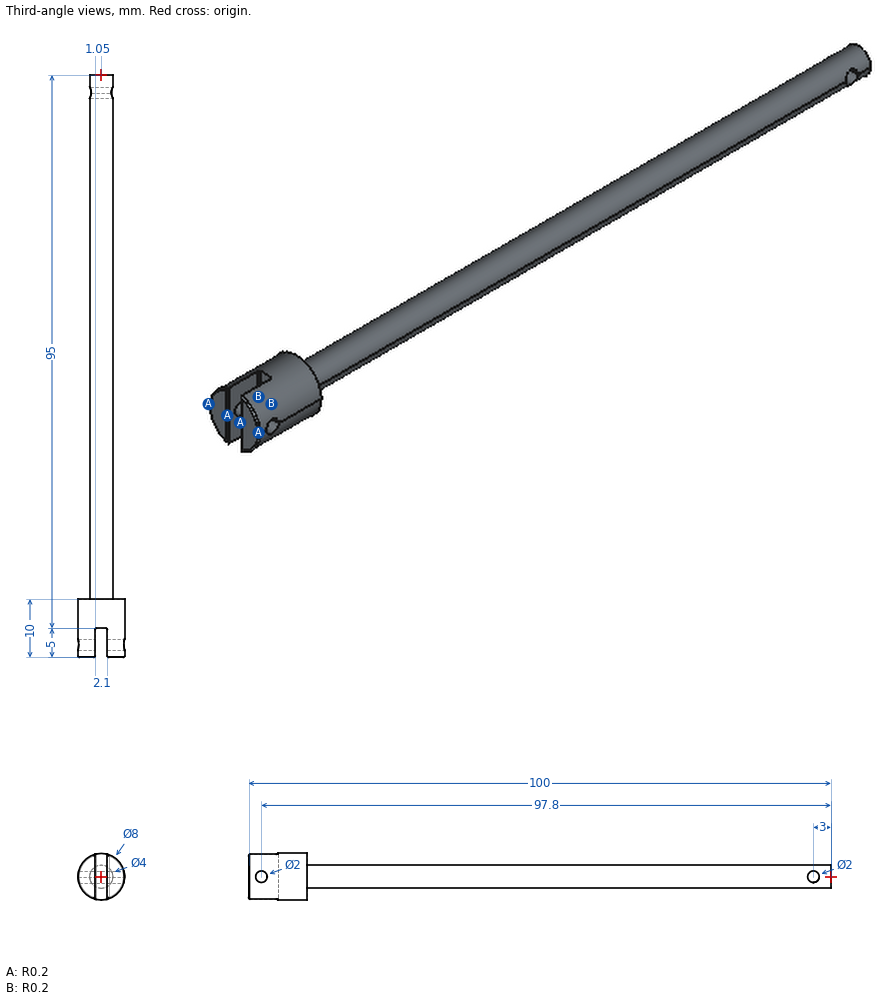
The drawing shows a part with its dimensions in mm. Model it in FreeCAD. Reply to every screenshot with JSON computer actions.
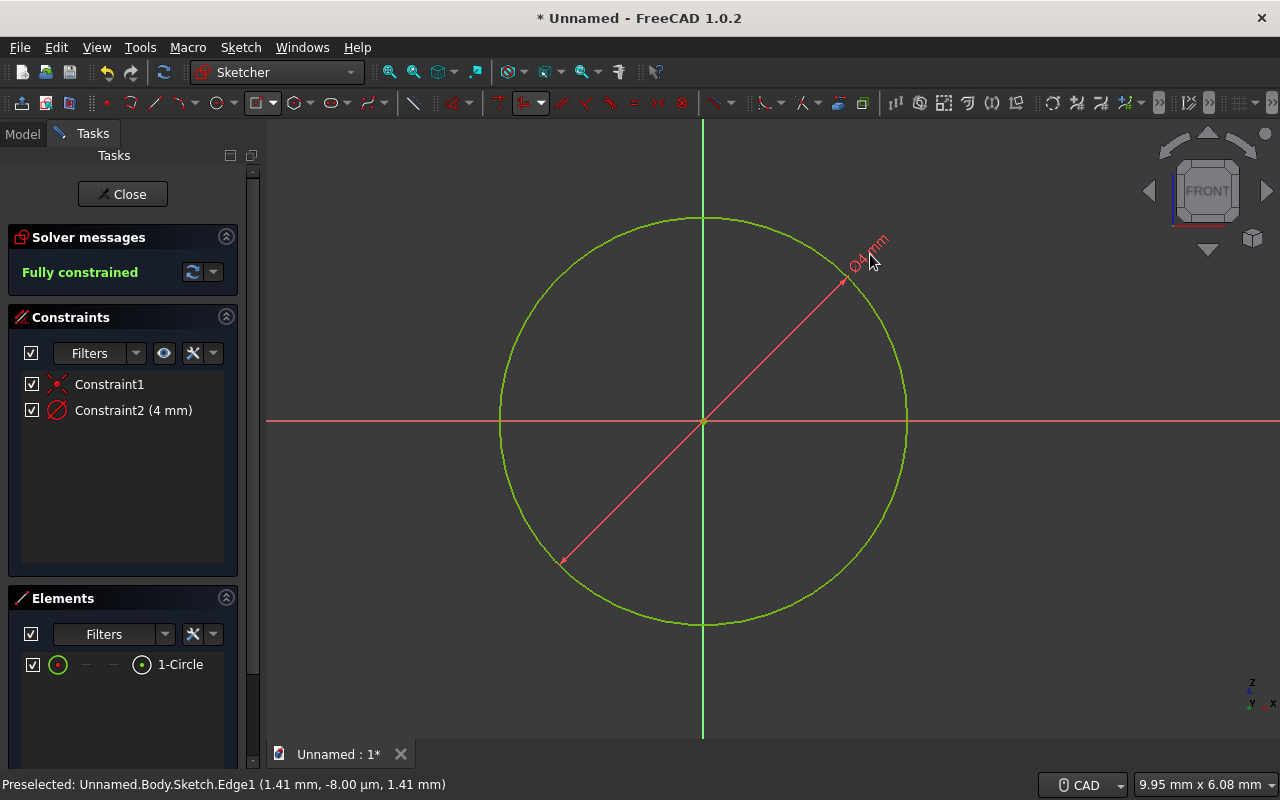
{"action": "left_click", "coordinate": [123, 194]}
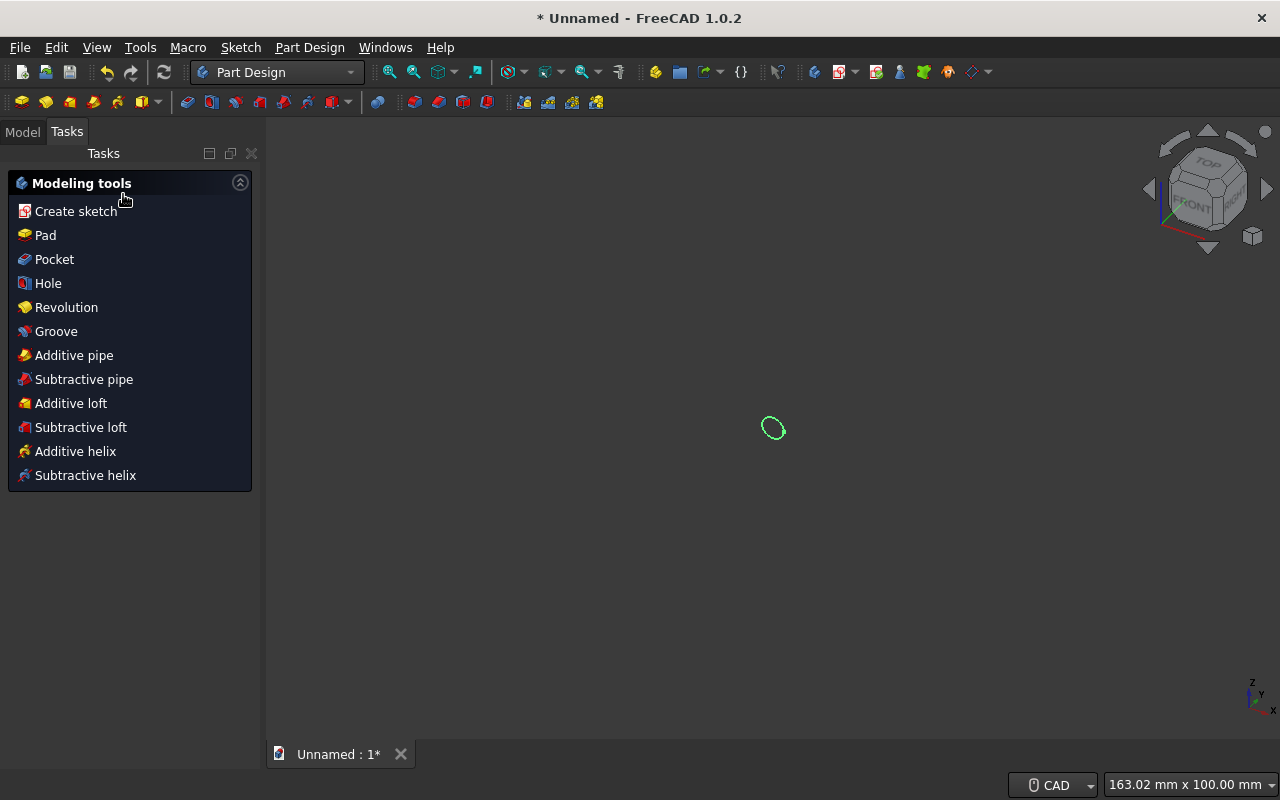
{"action": "left_click", "coordinate": [22, 102]}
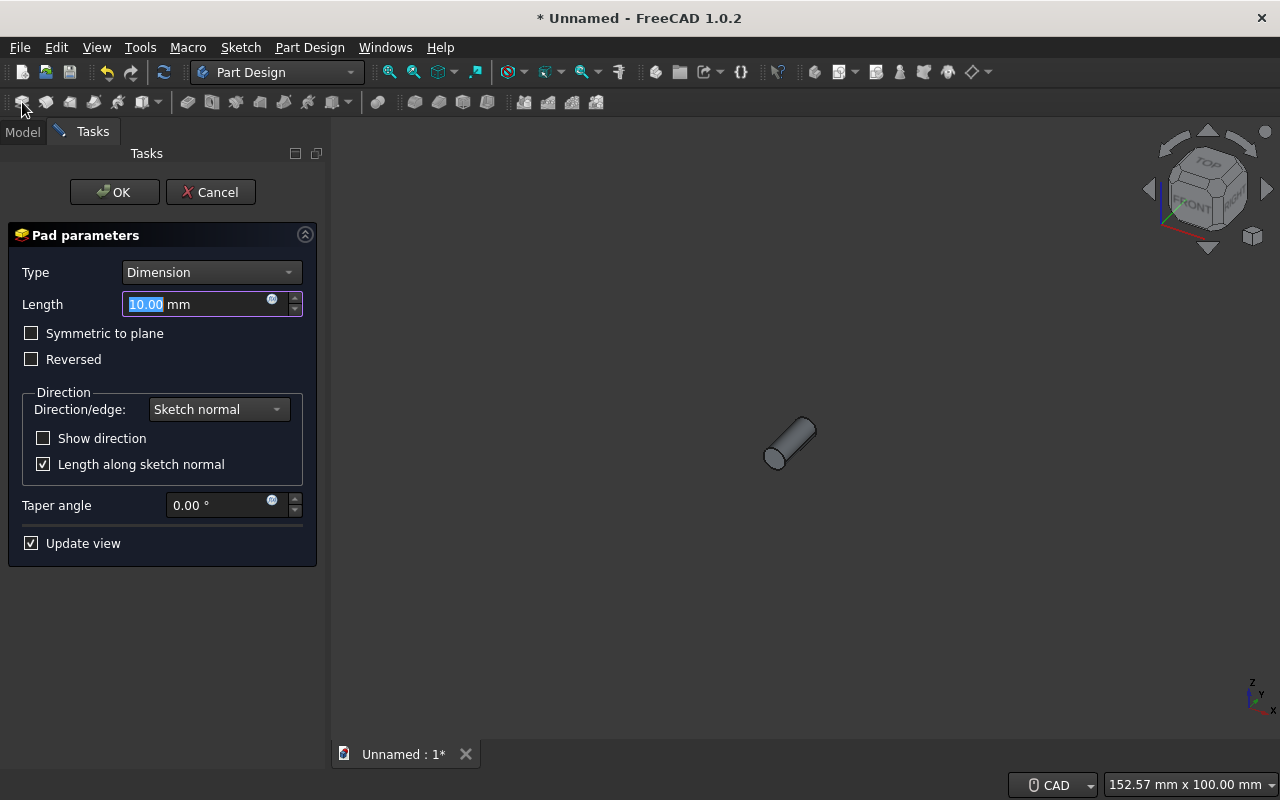
{"action": "type", "text": "100"}
{"action": "key", "text": "Tab"}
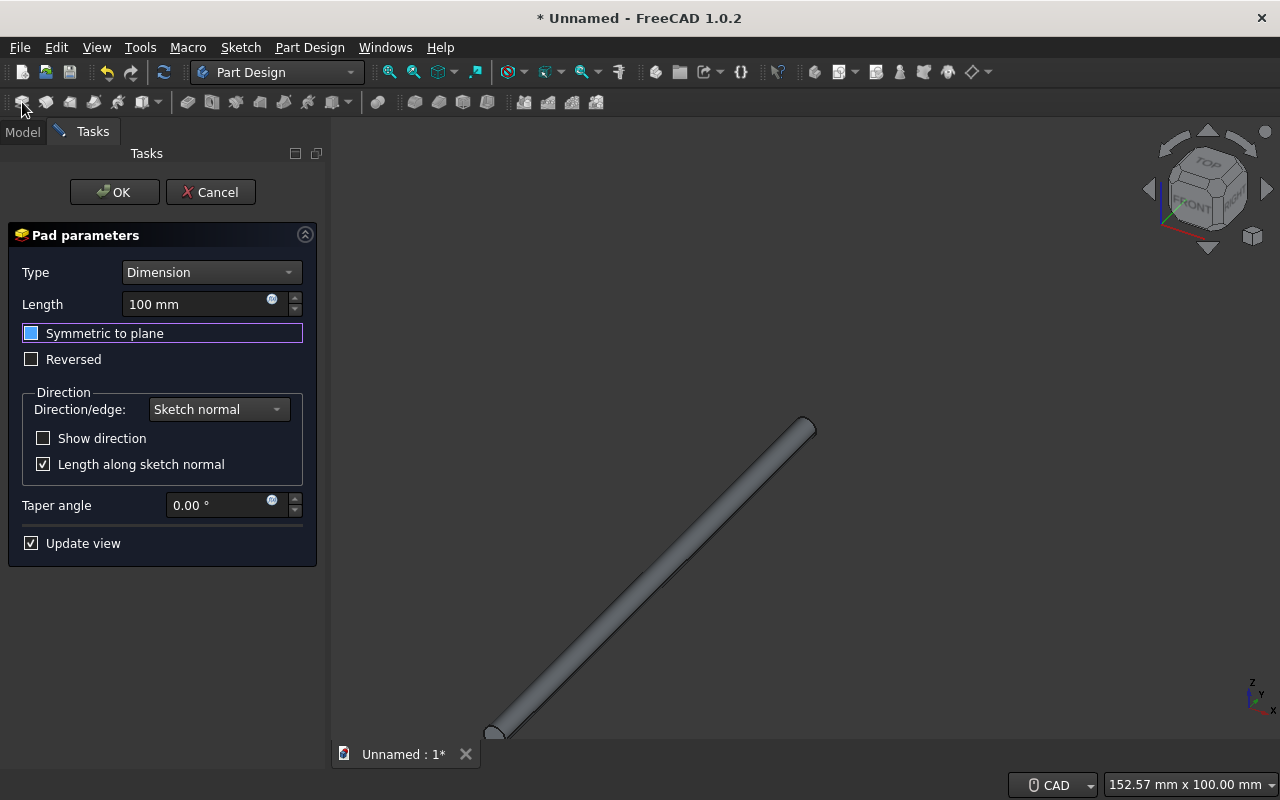
{"action": "left_click", "coordinate": [115, 192]}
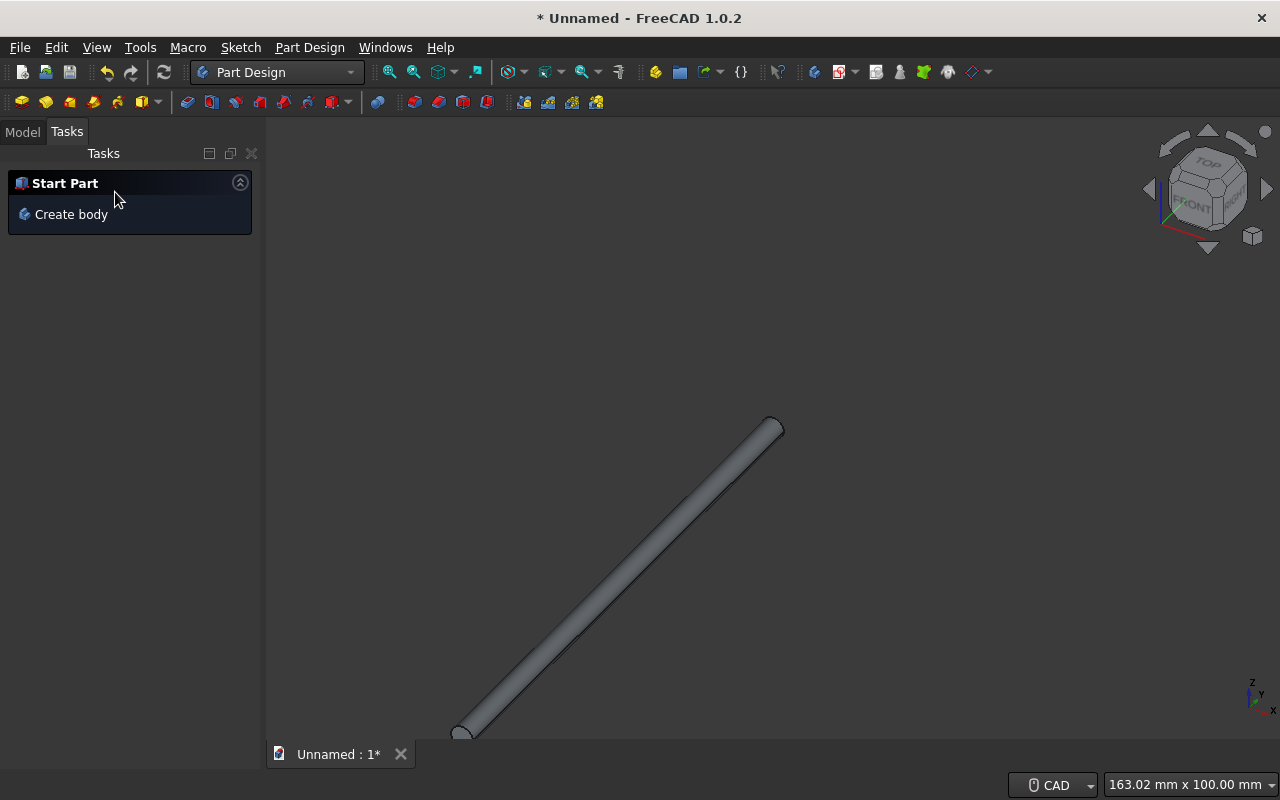
{"action": "left_click", "coordinate": [390, 72]}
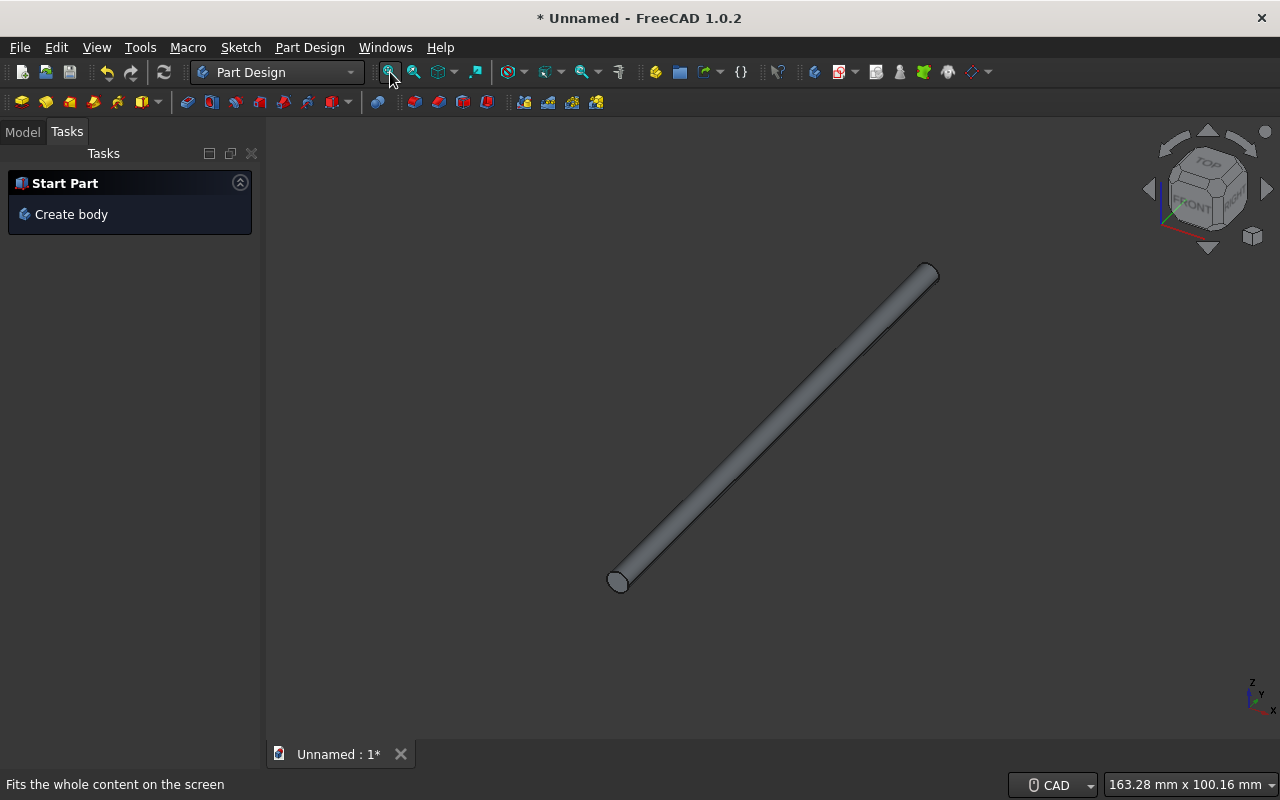
{"action": "left_click", "coordinate": [618, 584]}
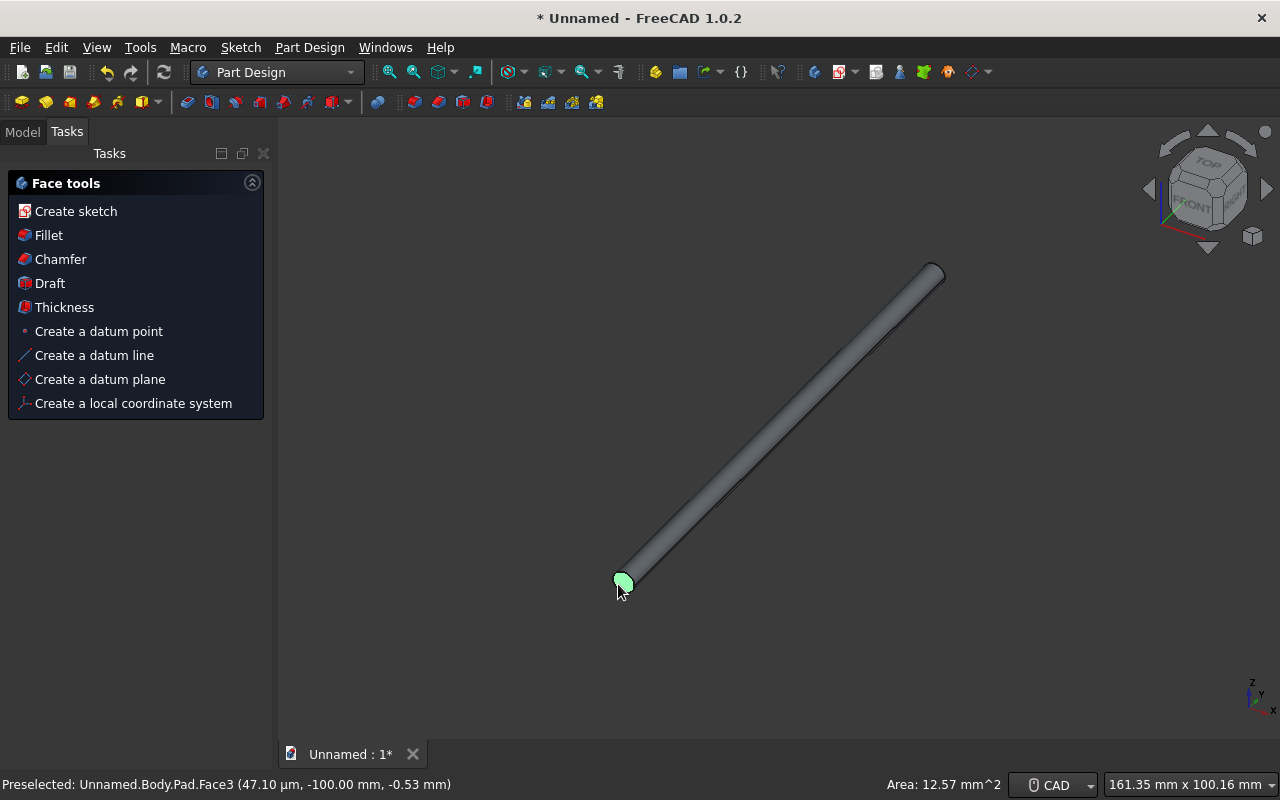
{"action": "left_click", "coordinate": [840, 72]}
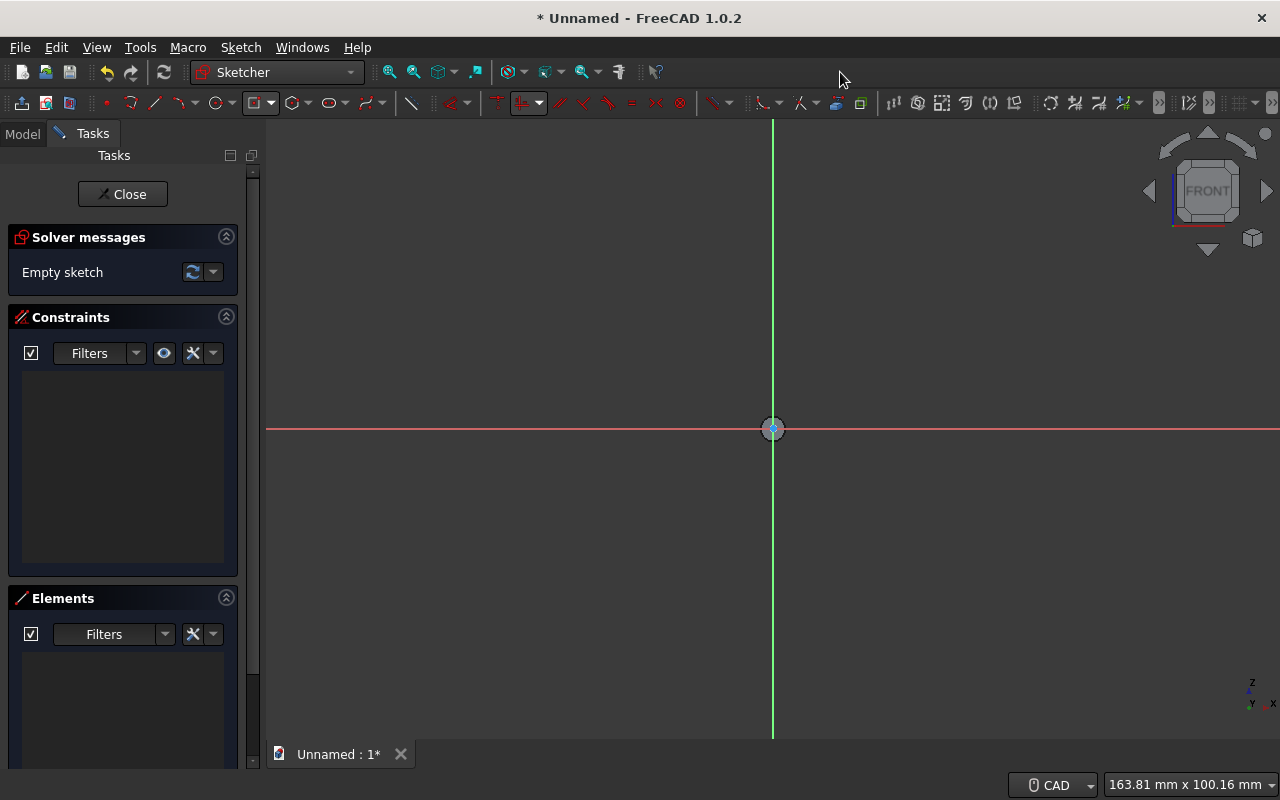
{"action": "scroll", "coordinate": [784, 429], "scroll_direction": "up", "scroll_amount": 10}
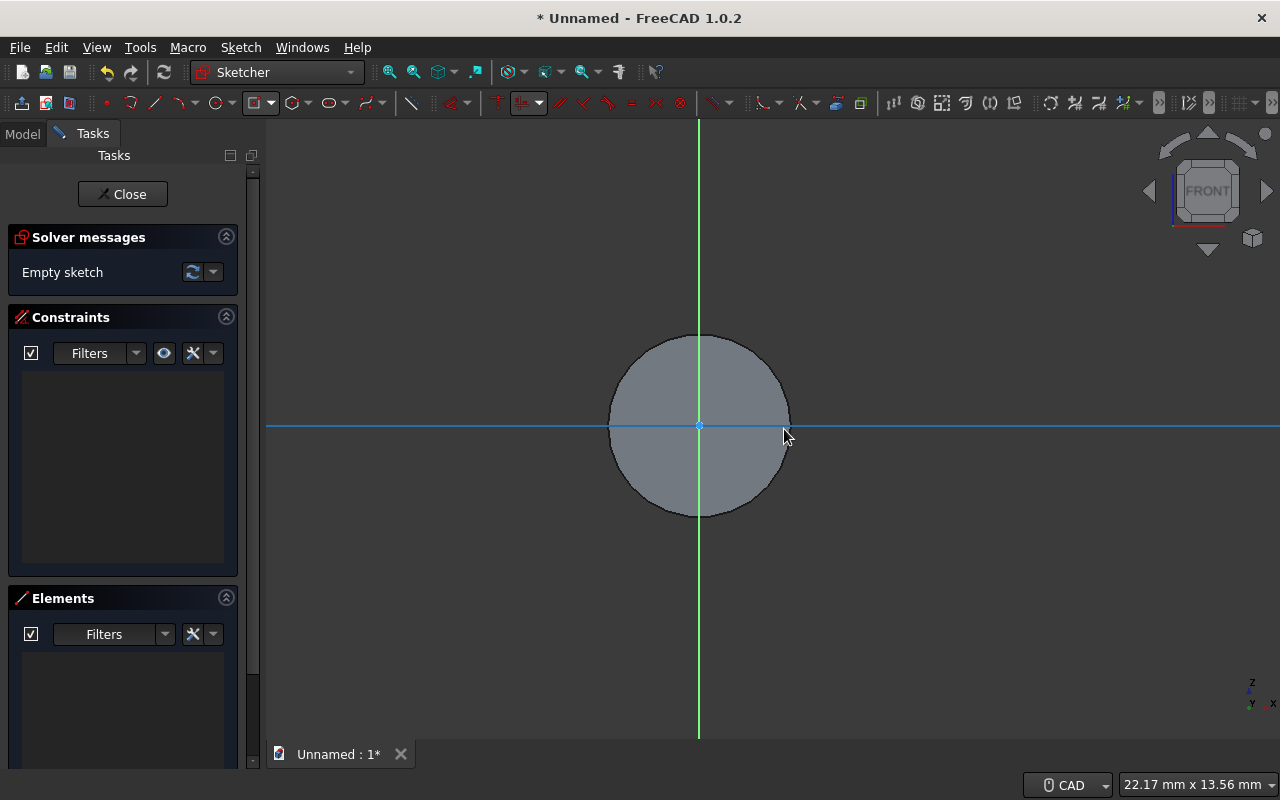
{"action": "left_click", "coordinate": [216, 104]}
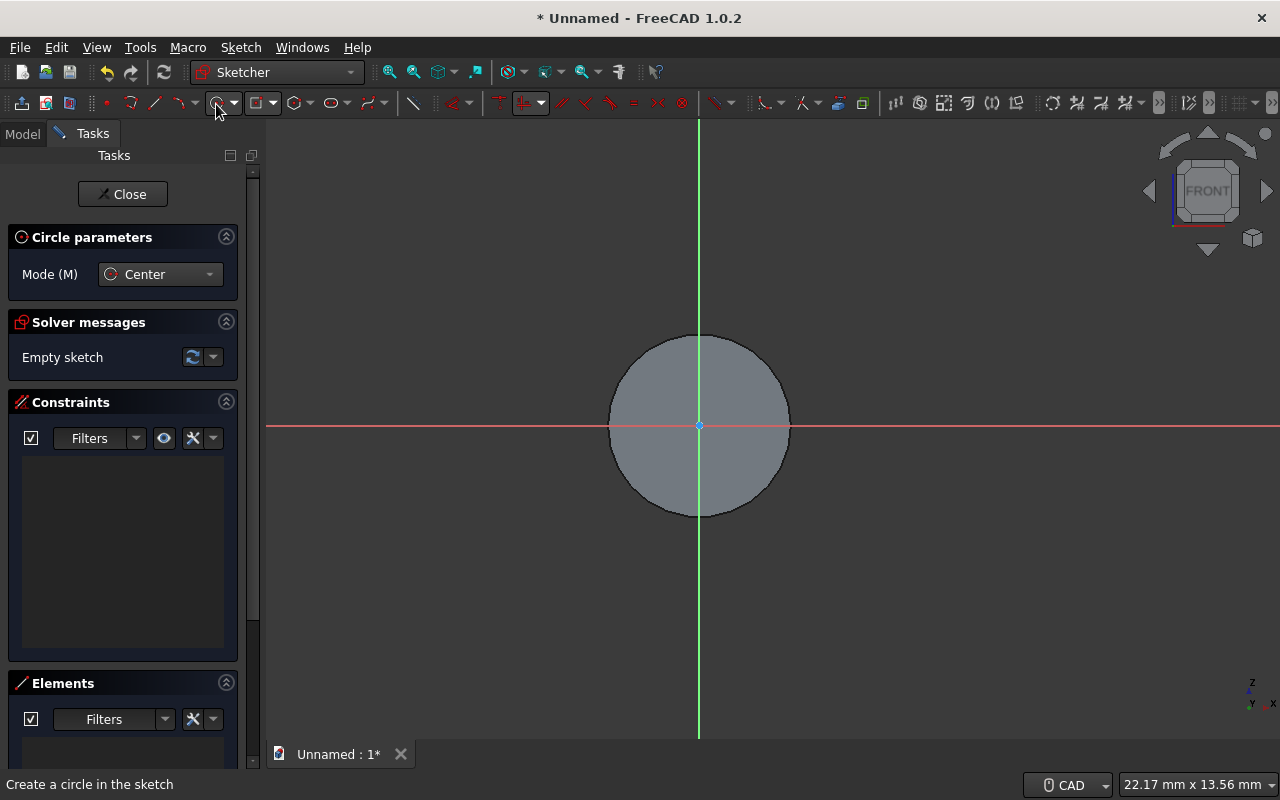
{"action": "left_click", "coordinate": [699, 426]}
{"action": "left_click", "coordinate": [829, 296]}
{"action": "key", "text": "Escape"}